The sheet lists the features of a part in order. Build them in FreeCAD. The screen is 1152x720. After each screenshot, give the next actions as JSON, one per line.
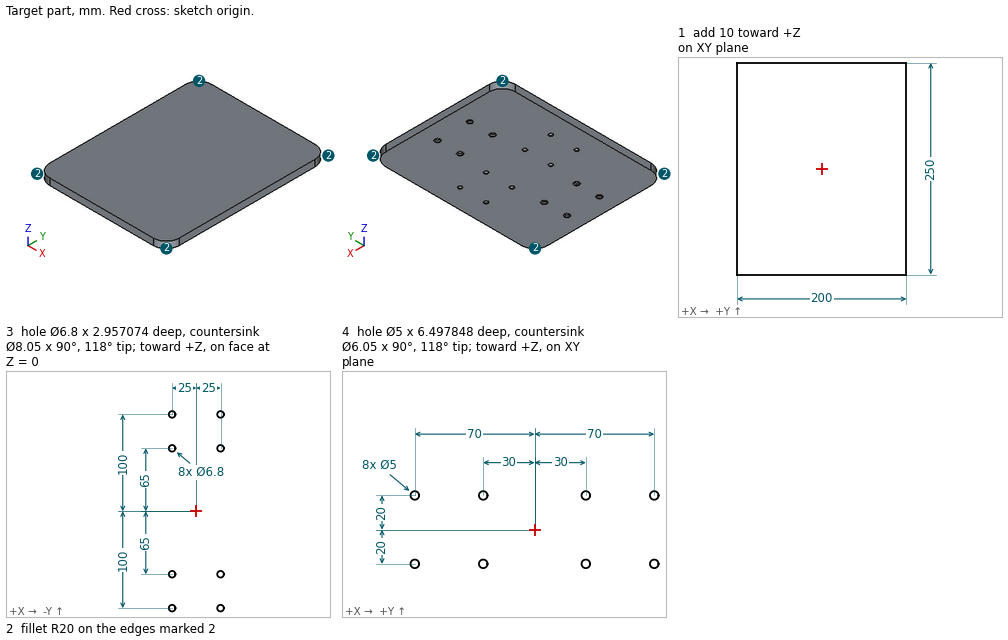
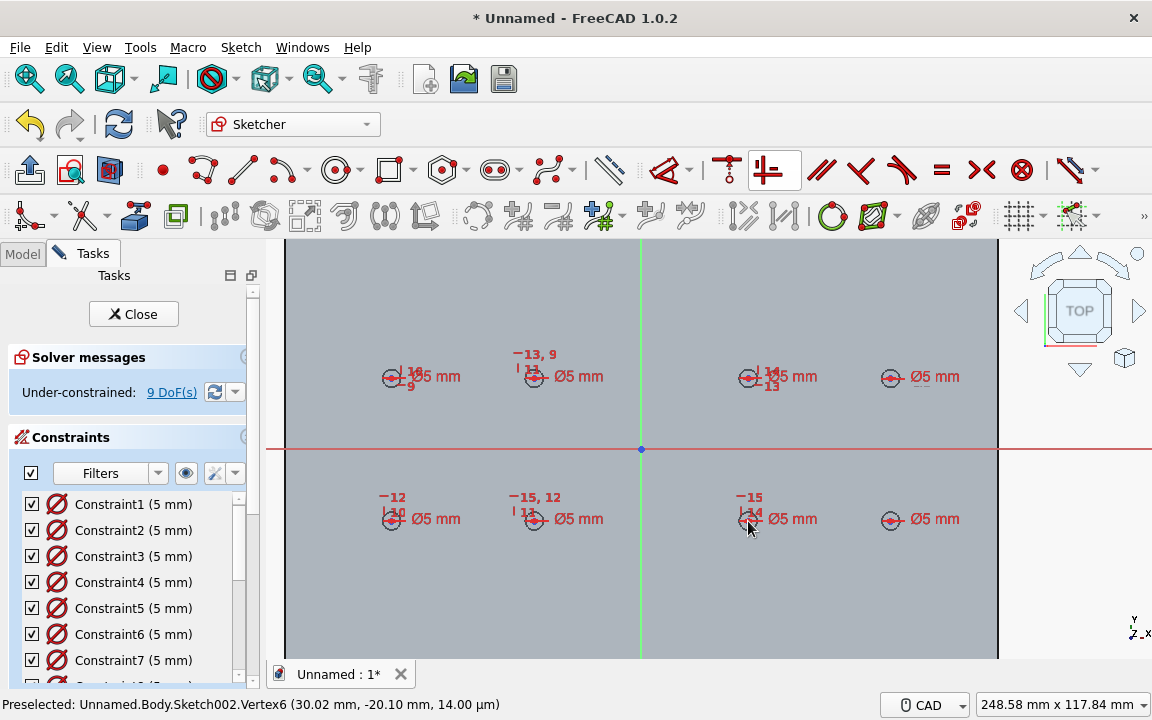
{"action": "left_click", "coordinate": [748, 378]}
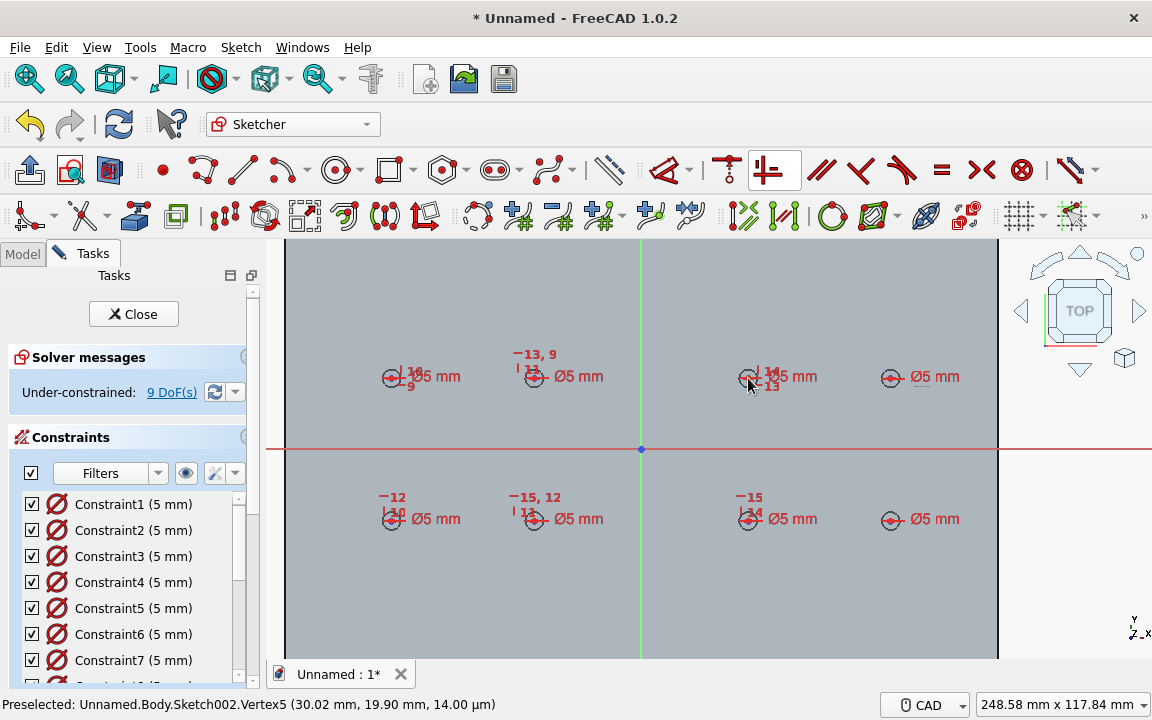
{"action": "left_click", "coordinate": [891, 379]}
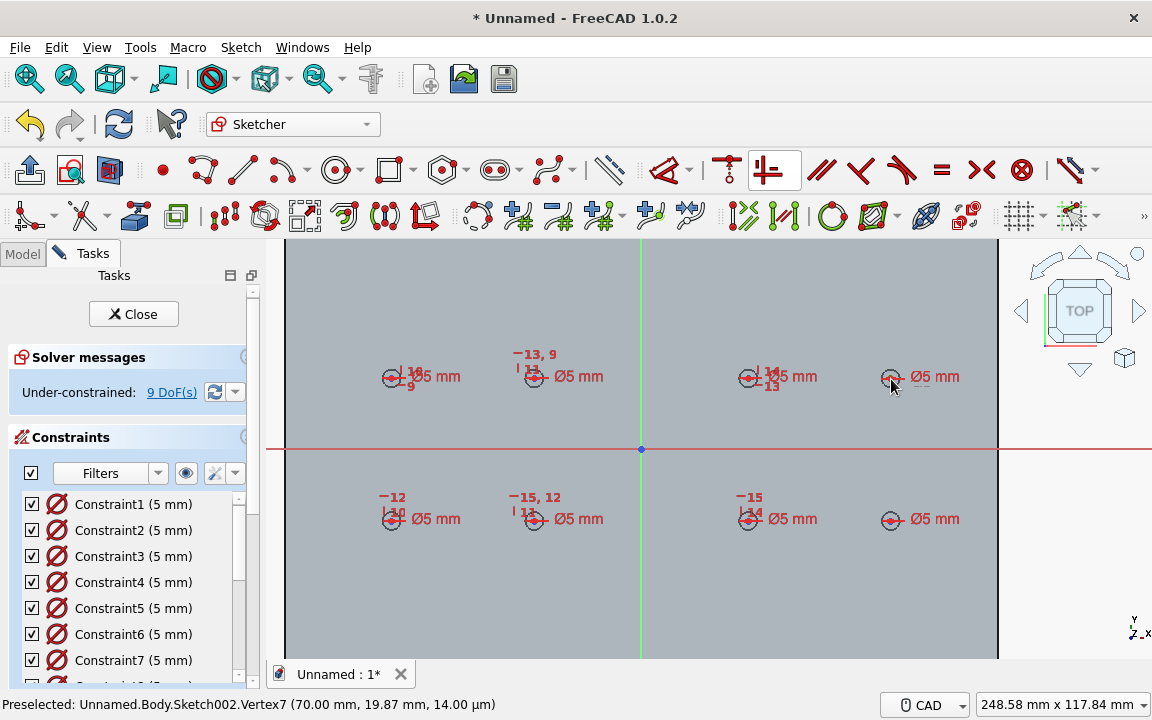
{"action": "key", "text": "h"}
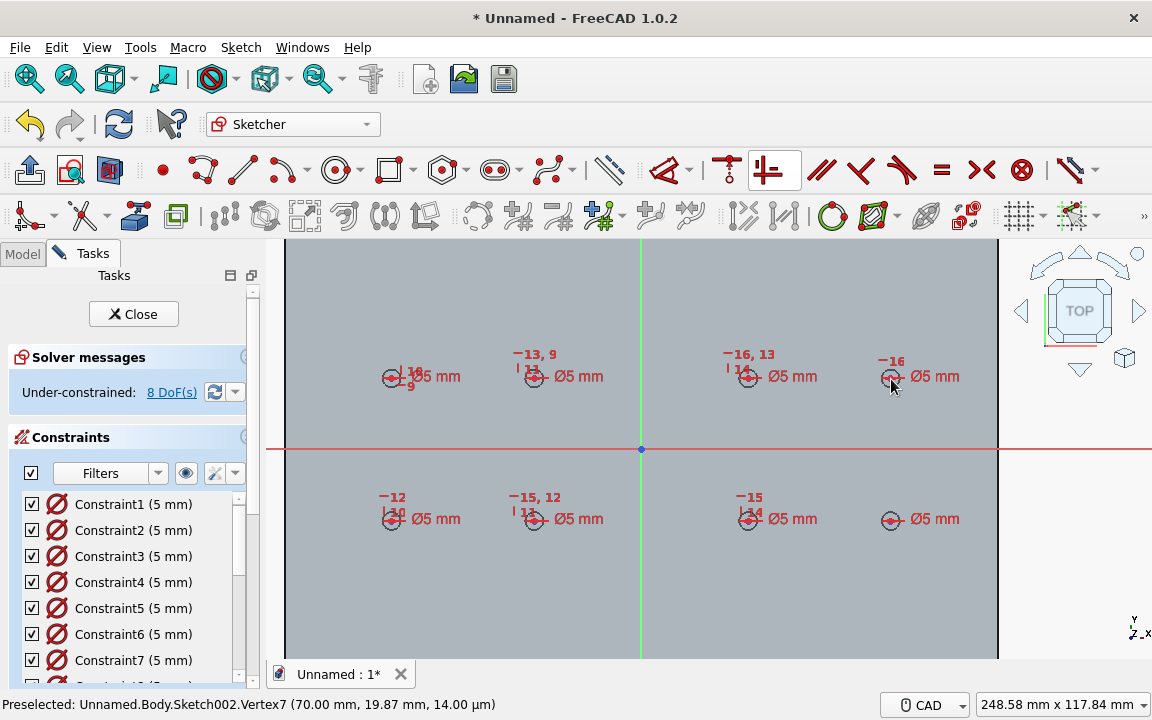
{"action": "left_click", "coordinate": [891, 378]}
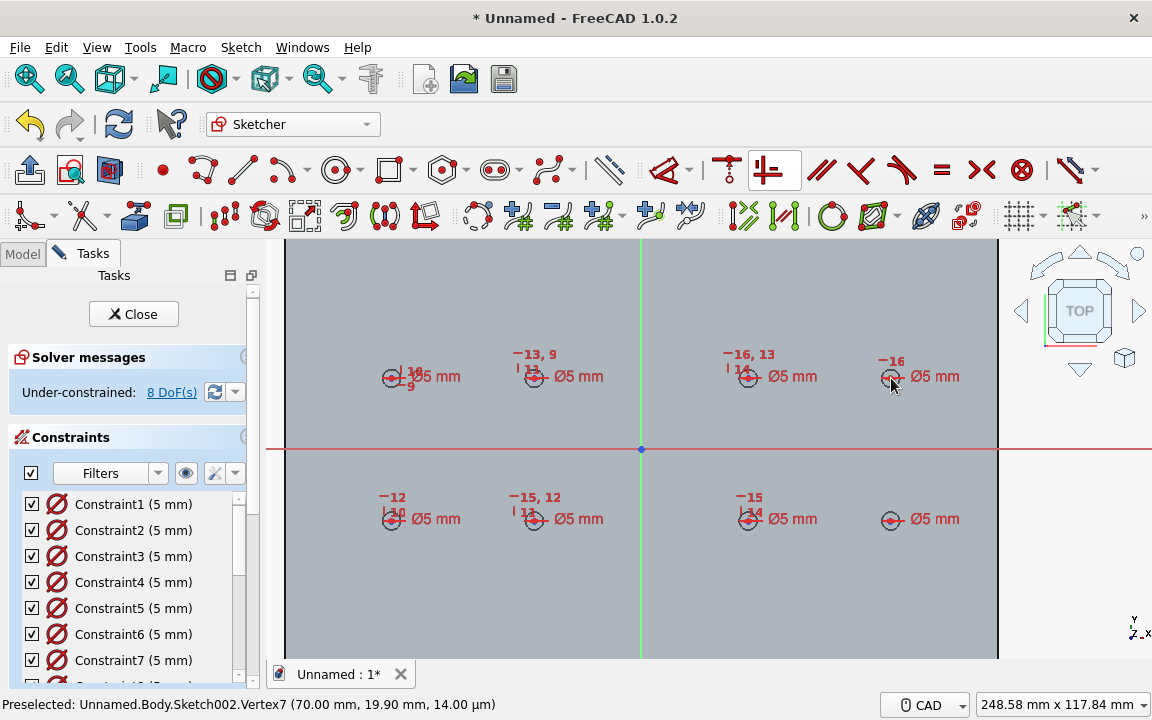
{"action": "left_click", "coordinate": [891, 521]}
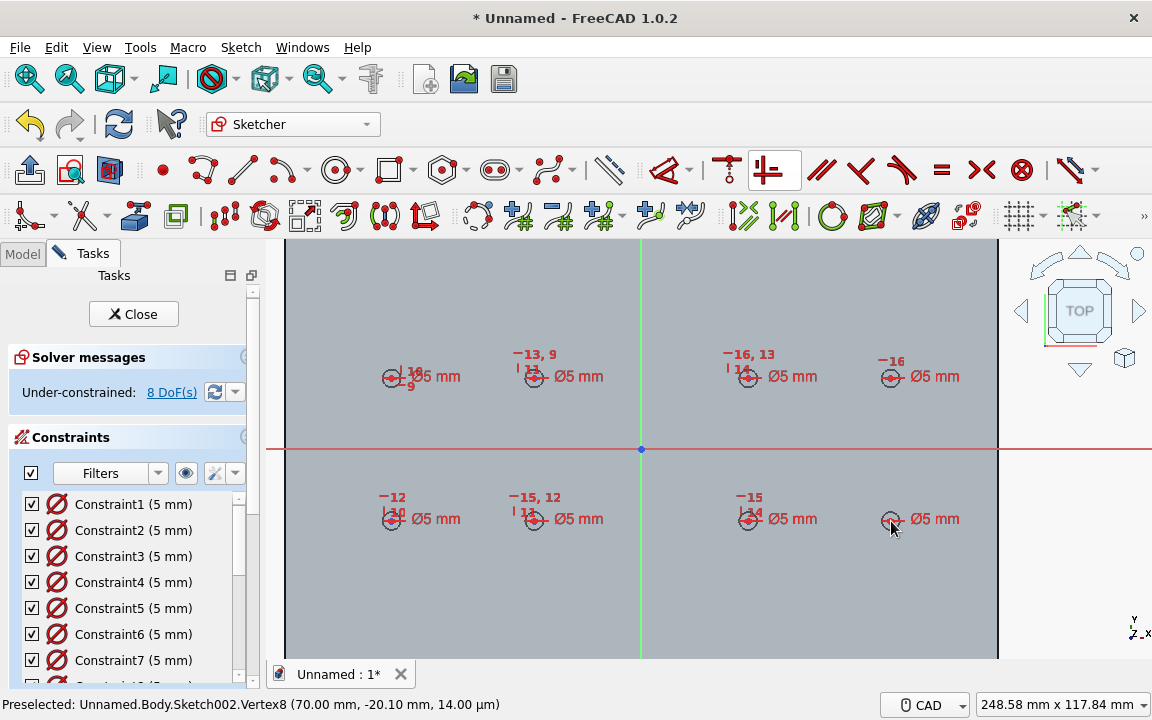
{"action": "key", "text": "v"}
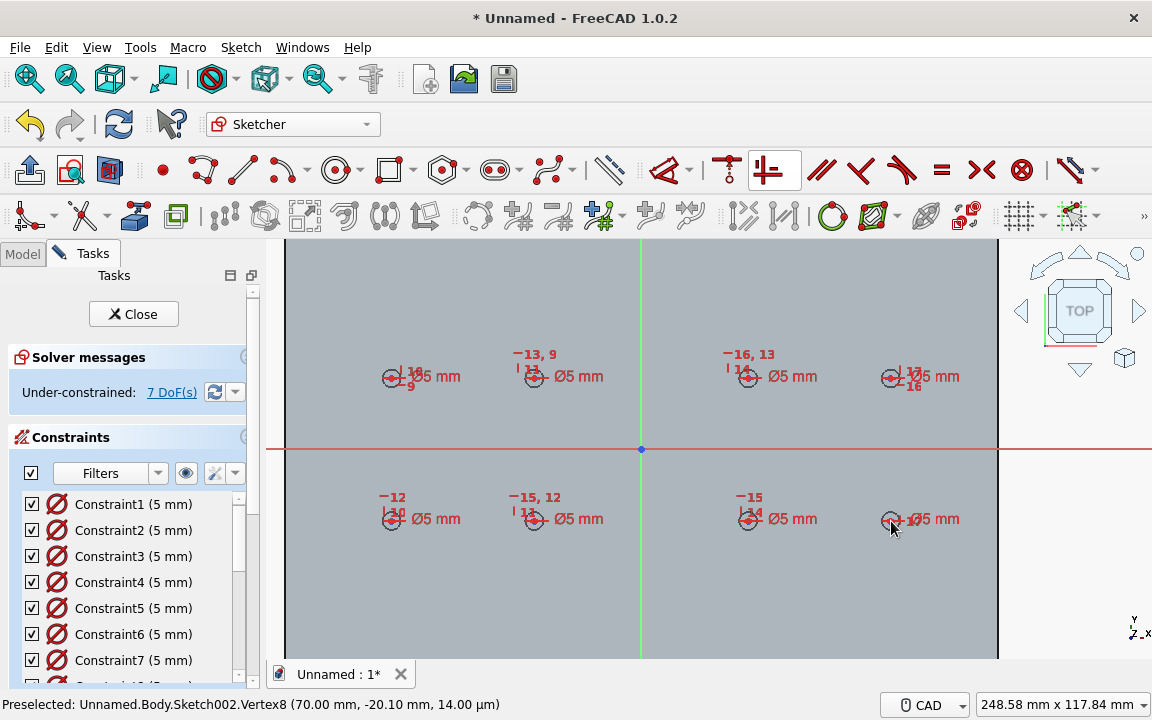
{"action": "left_click", "coordinate": [748, 521]}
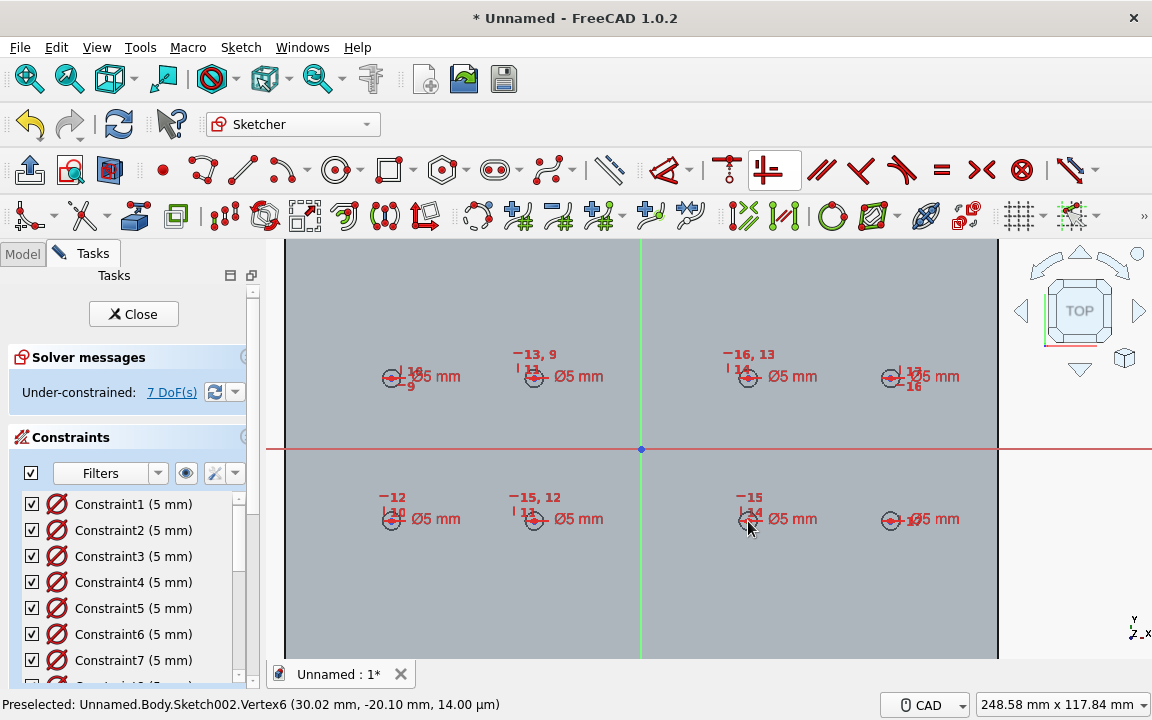
{"action": "left_click", "coordinate": [891, 521]}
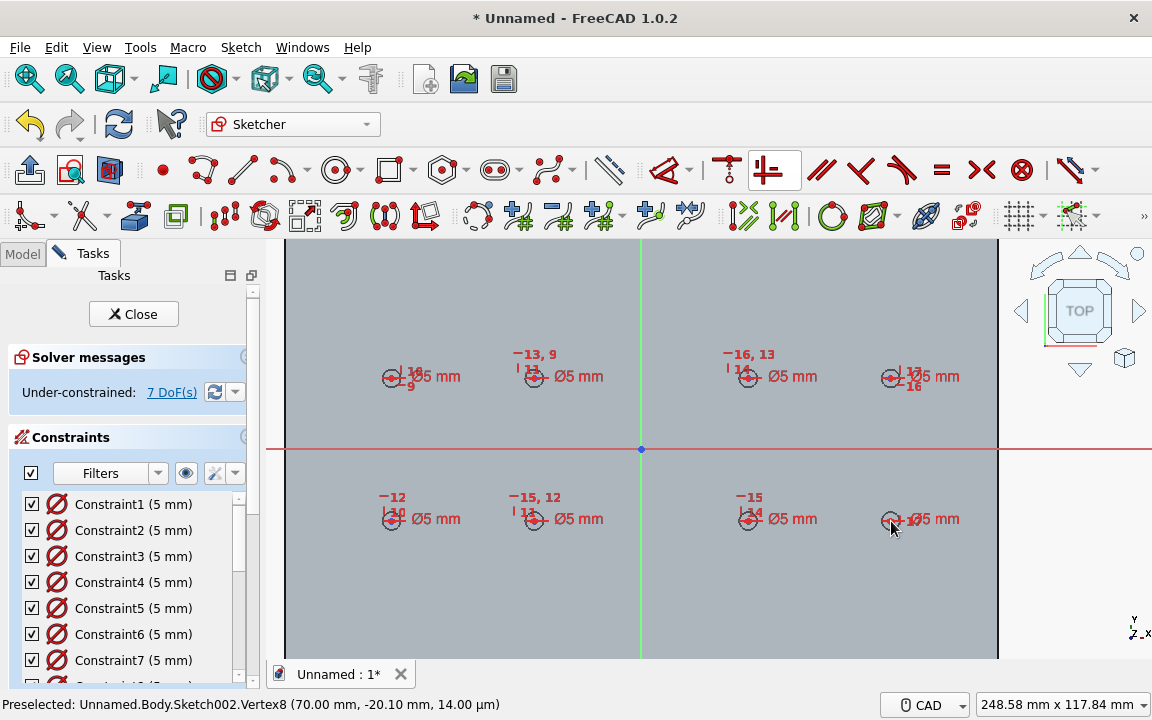
{"action": "key", "text": "h"}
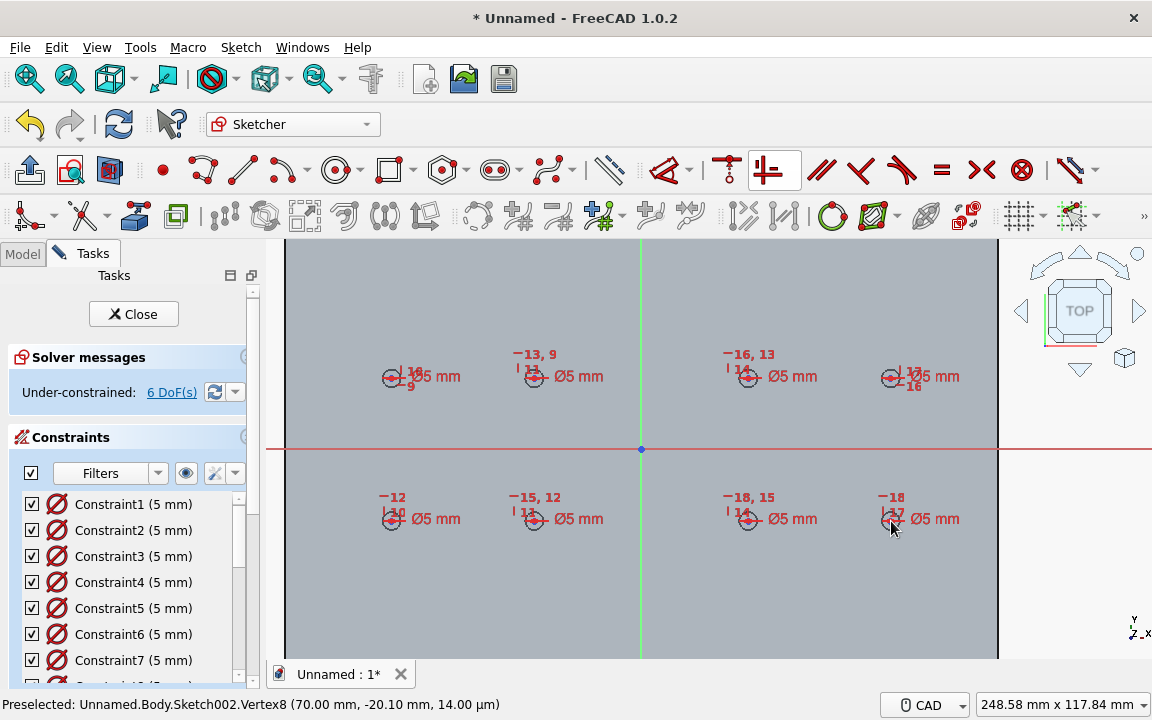
{"action": "left_click", "coordinate": [664, 170]}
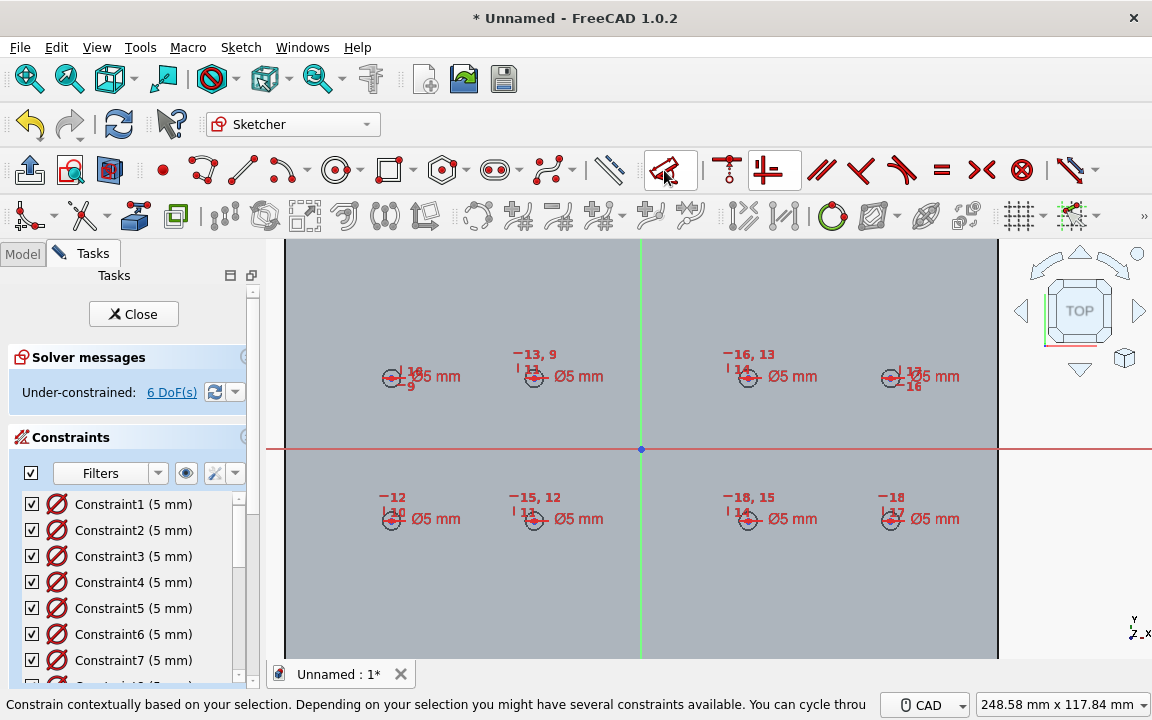
{"action": "left_click", "coordinate": [392, 378]}
{"action": "left_click", "coordinate": [516, 344]}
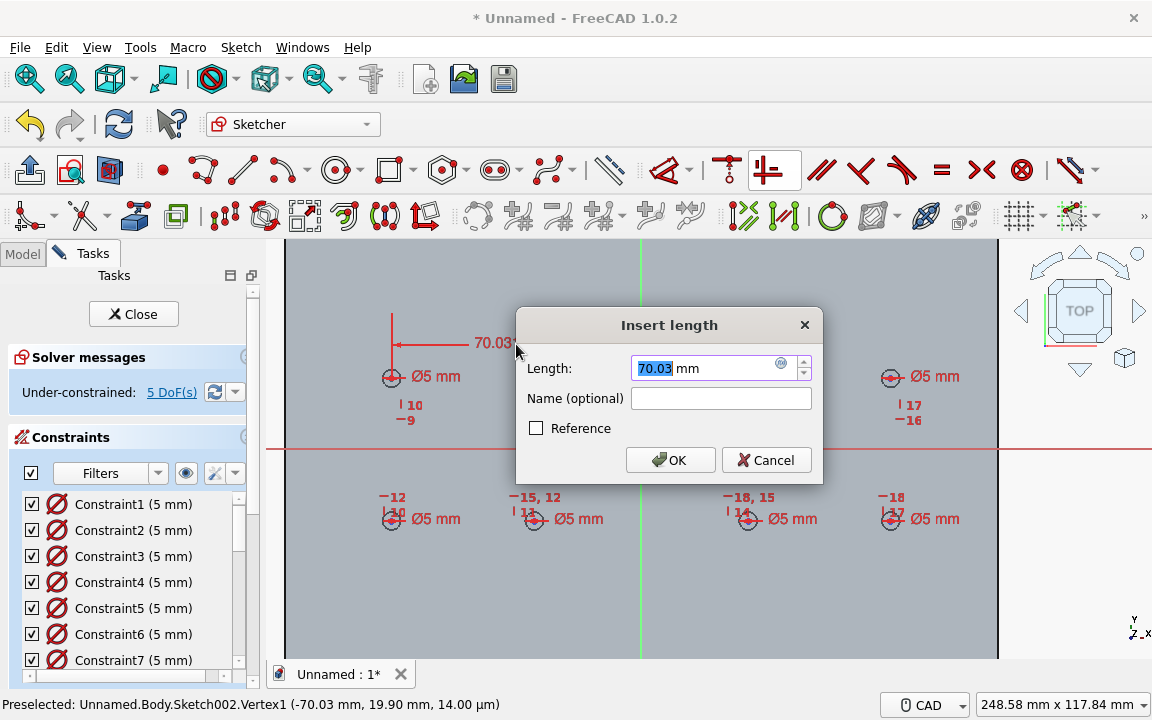
{"action": "type", "text": "70"}
{"action": "key", "text": "Return"}